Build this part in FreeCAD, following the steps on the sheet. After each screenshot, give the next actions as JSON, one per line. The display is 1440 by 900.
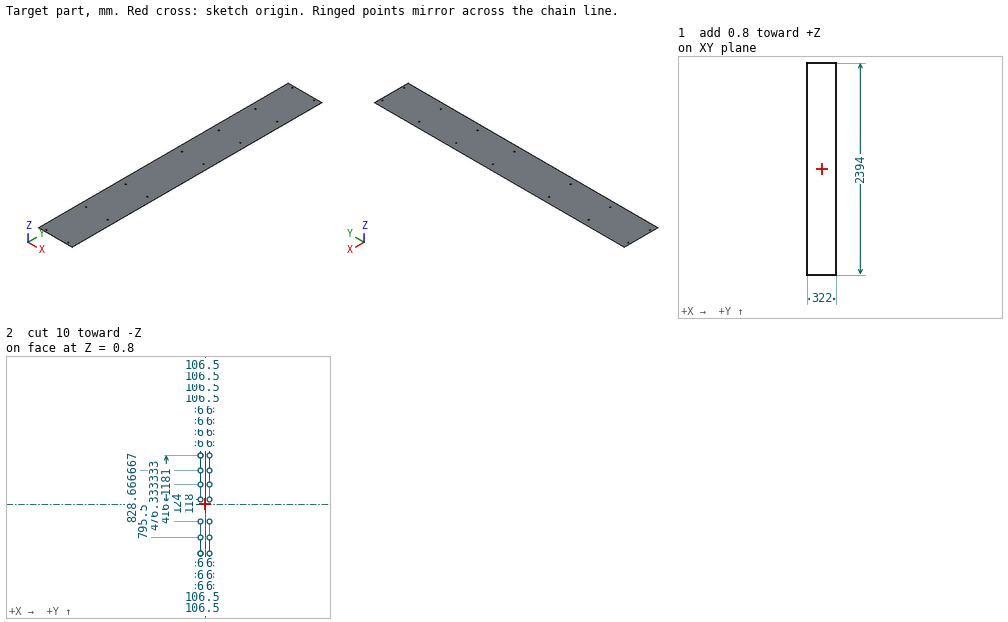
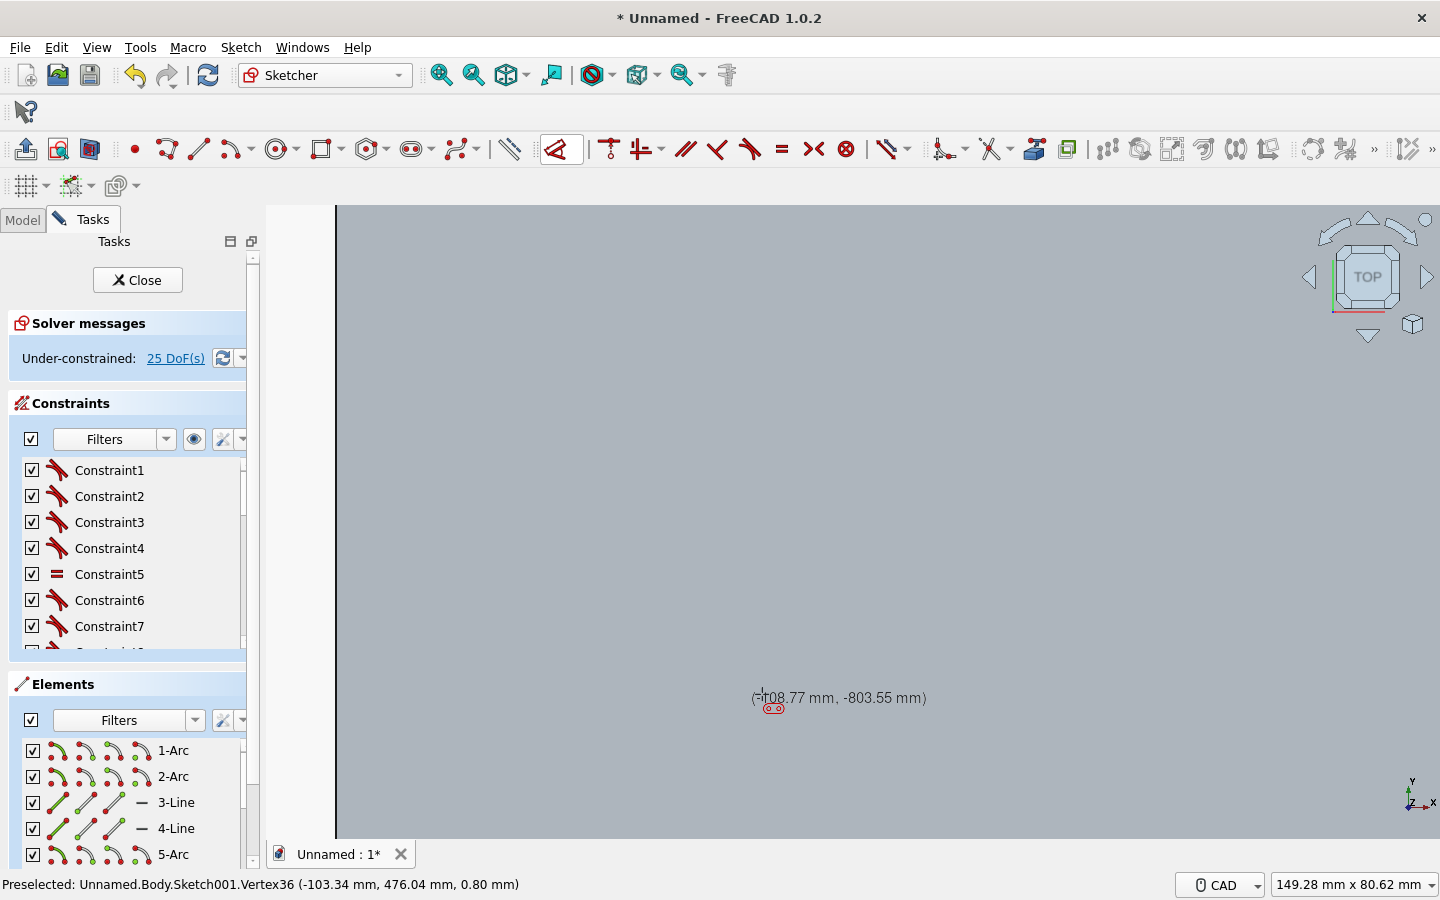
{"action": "scroll", "coordinate": [762, 694], "scroll_direction": "down", "scroll_amount": 18}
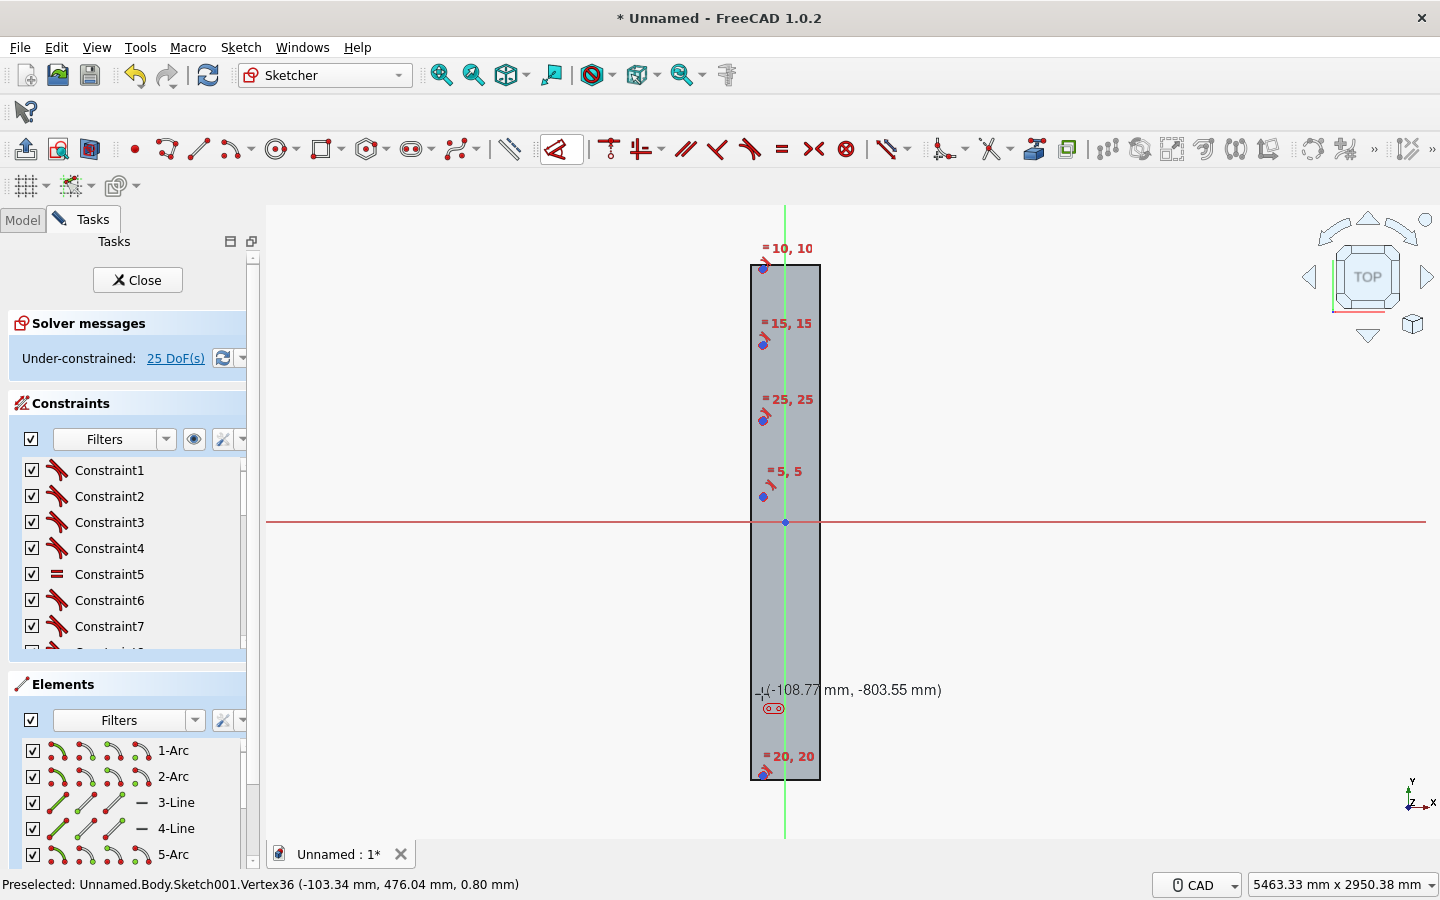
{"action": "left_click", "coordinate": [762, 694]}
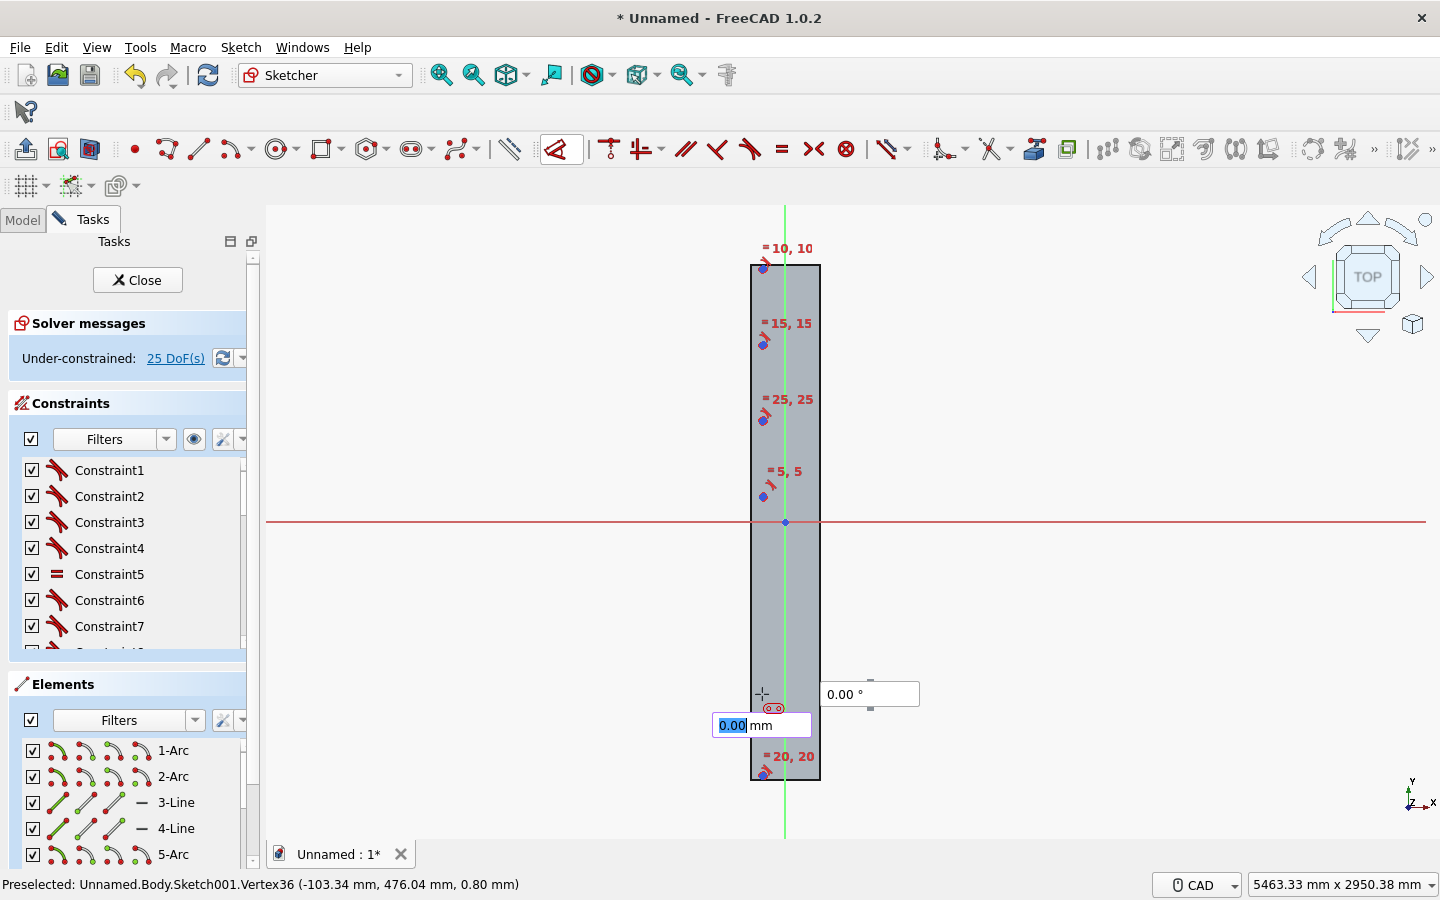
{"action": "scroll", "coordinate": [764, 694], "scroll_direction": "up", "scroll_amount": 13}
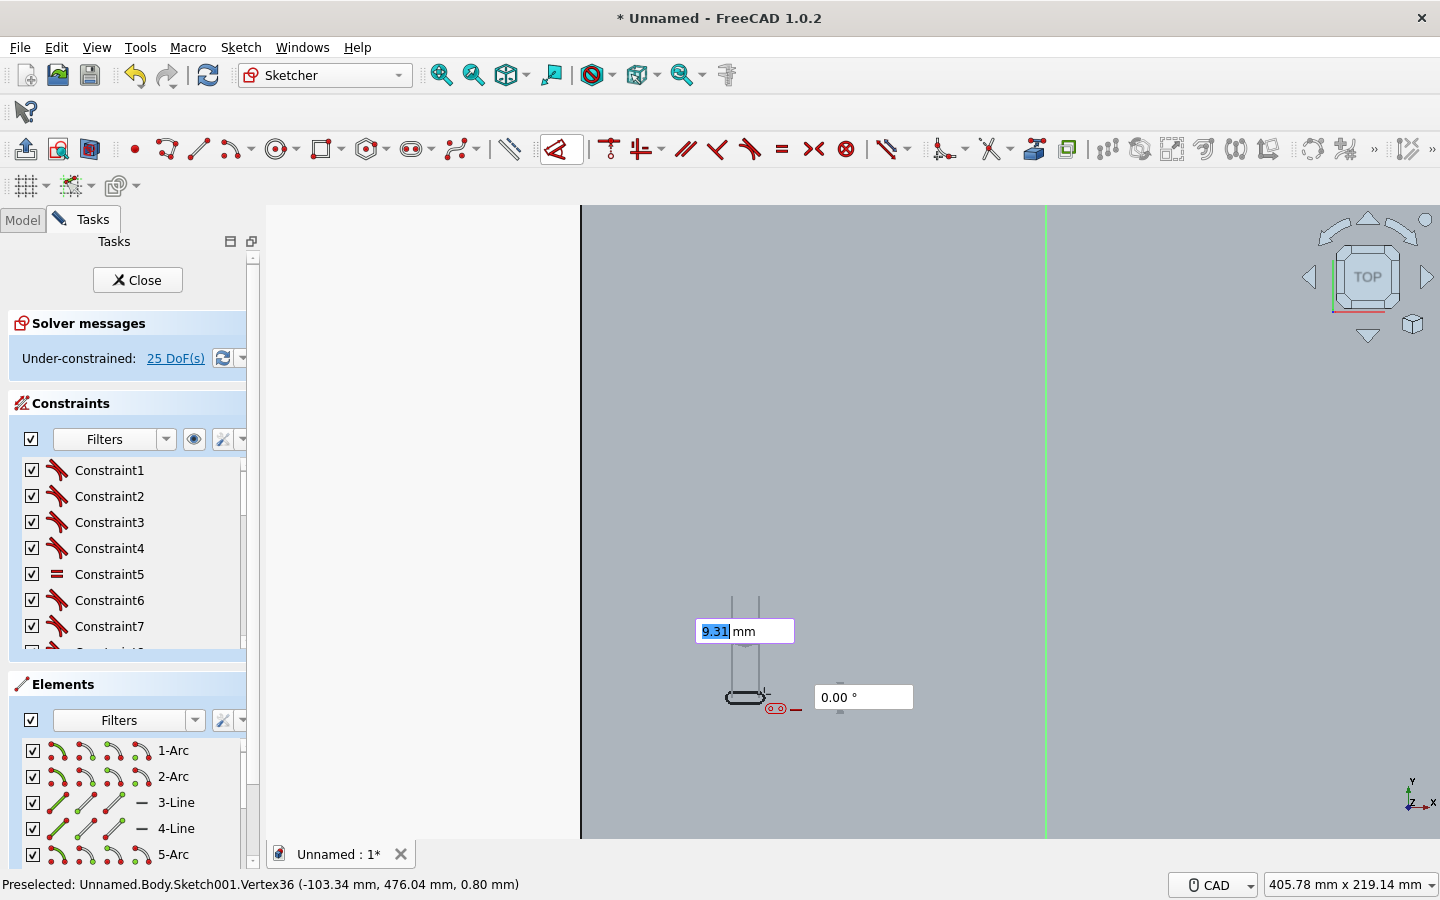
{"action": "left_click", "coordinate": [756, 684]}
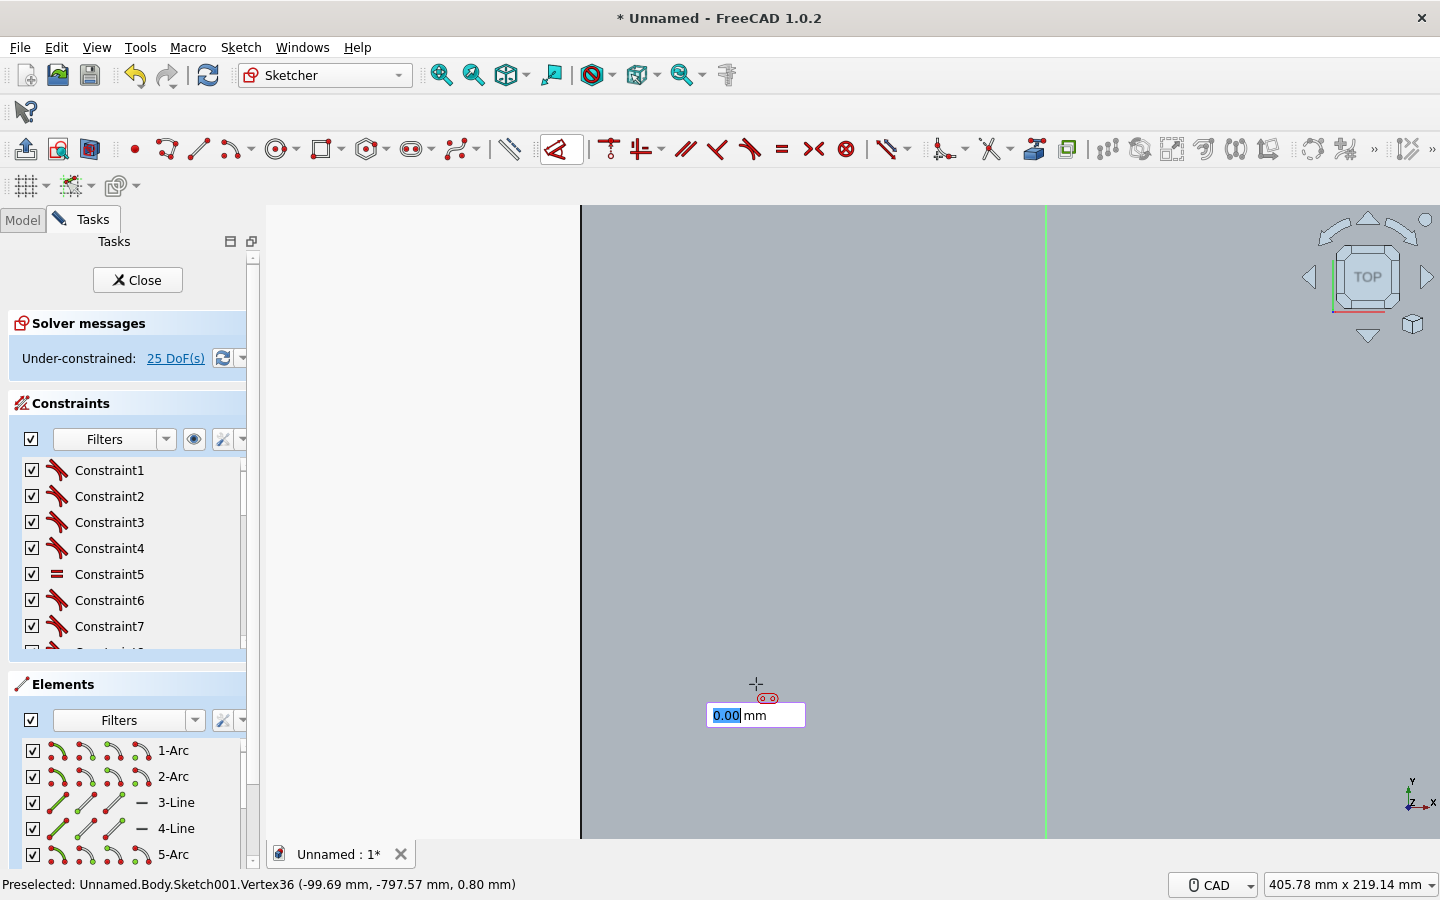
{"action": "scroll", "coordinate": [747, 675], "scroll_direction": "up", "scroll_amount": 4}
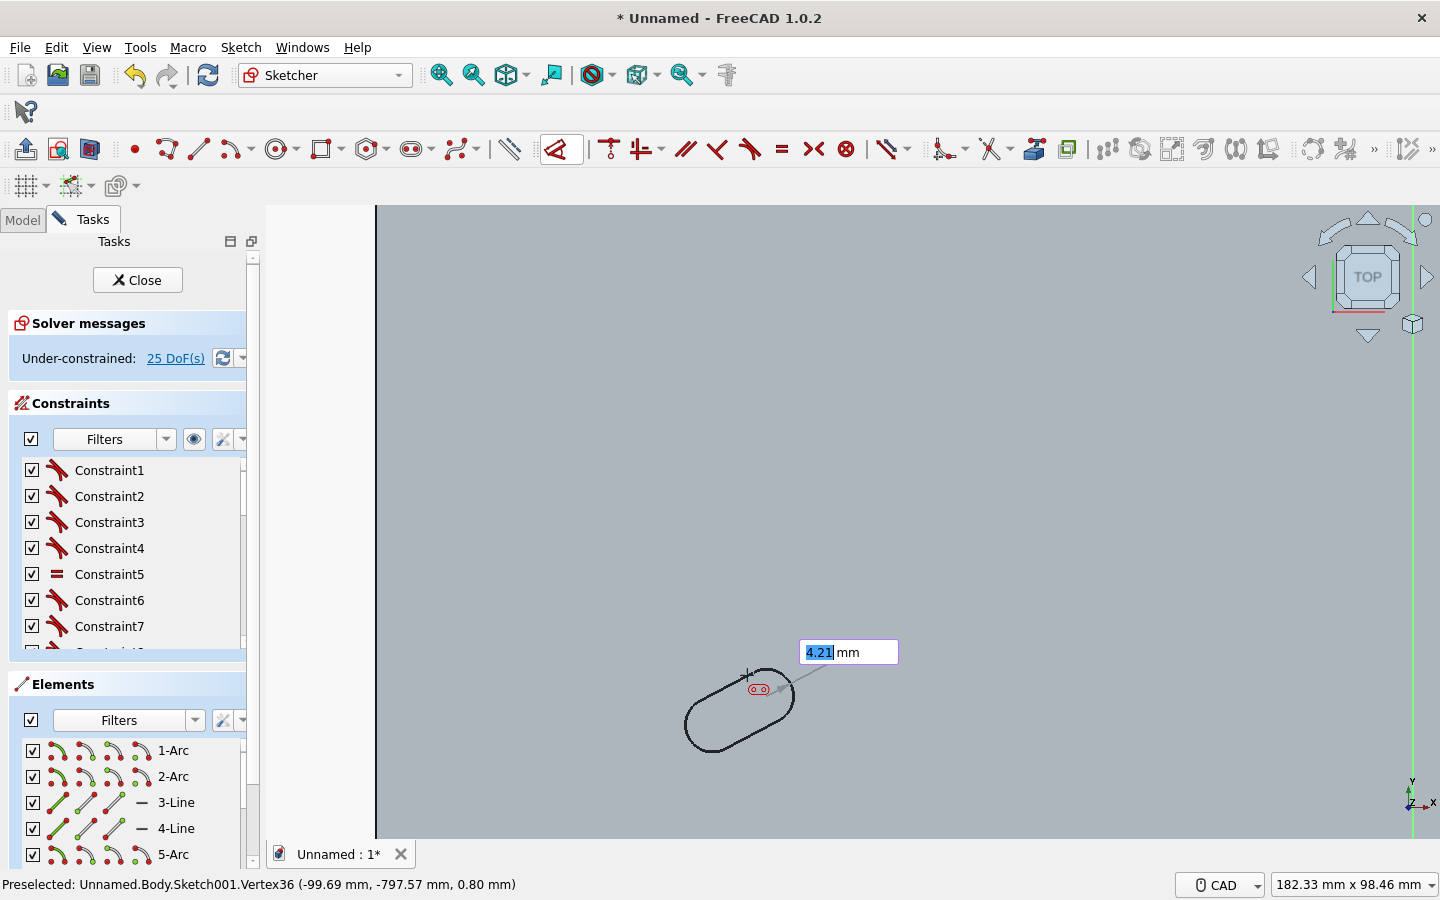
{"action": "left_click", "coordinate": [747, 673]}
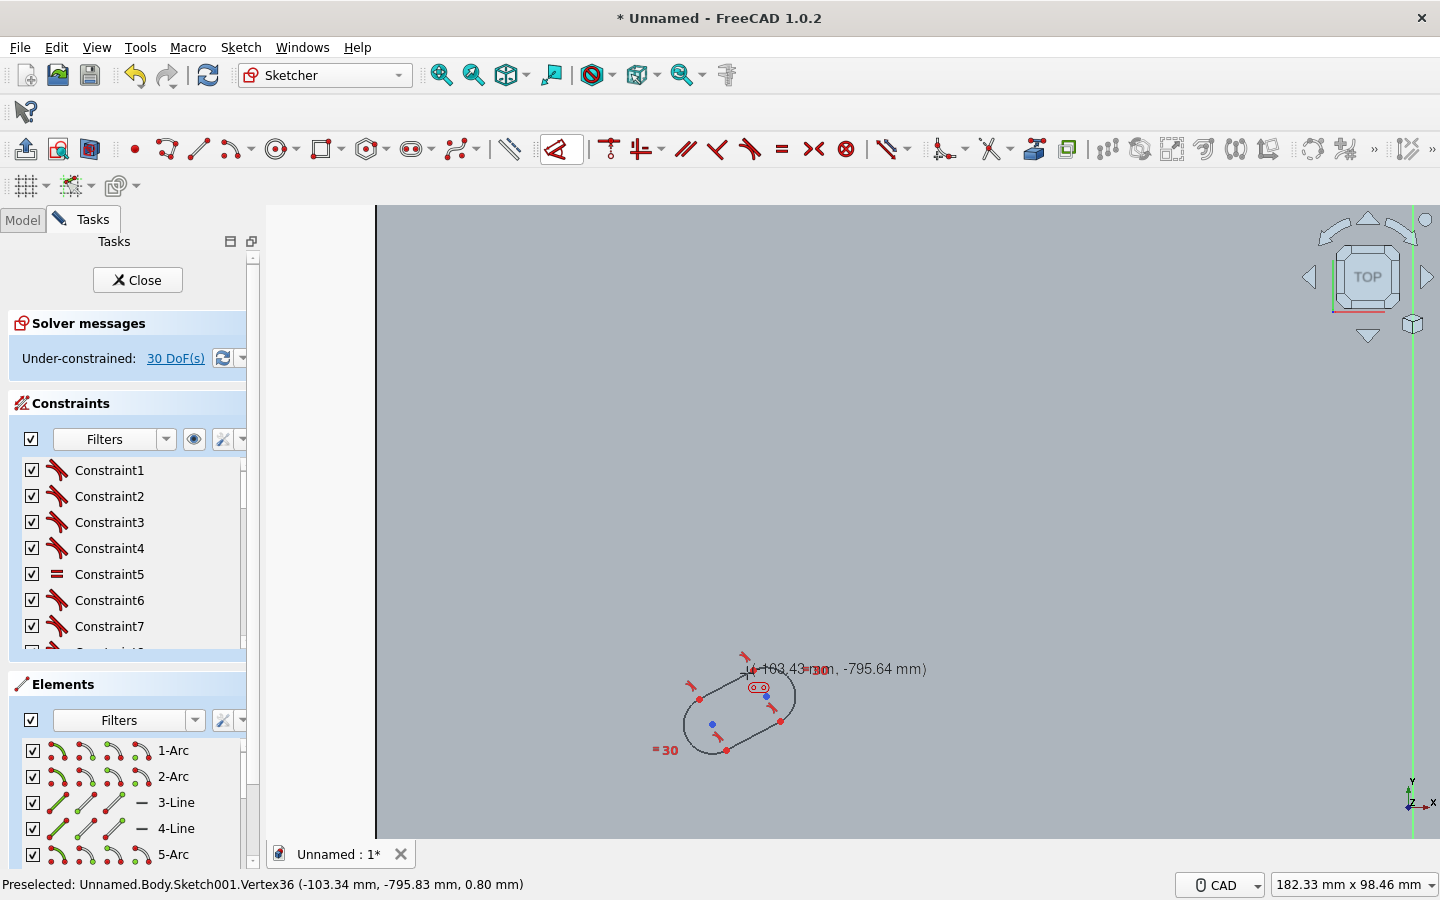
{"action": "scroll", "coordinate": [763, 694], "scroll_direction": "down", "scroll_amount": 17}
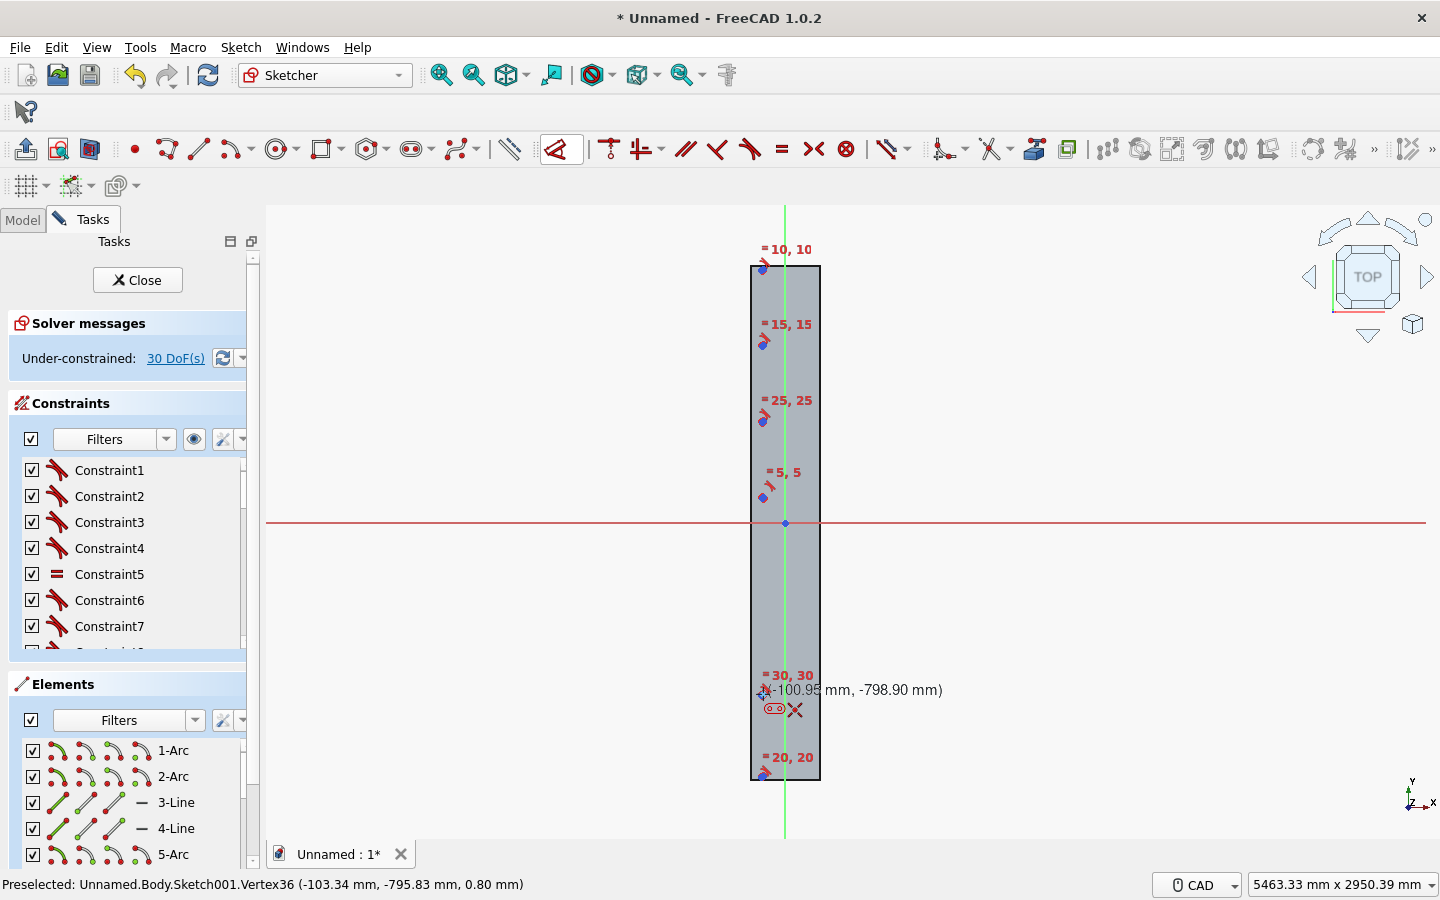
{"action": "scroll", "coordinate": [762, 613], "scroll_direction": "up", "scroll_amount": 18}